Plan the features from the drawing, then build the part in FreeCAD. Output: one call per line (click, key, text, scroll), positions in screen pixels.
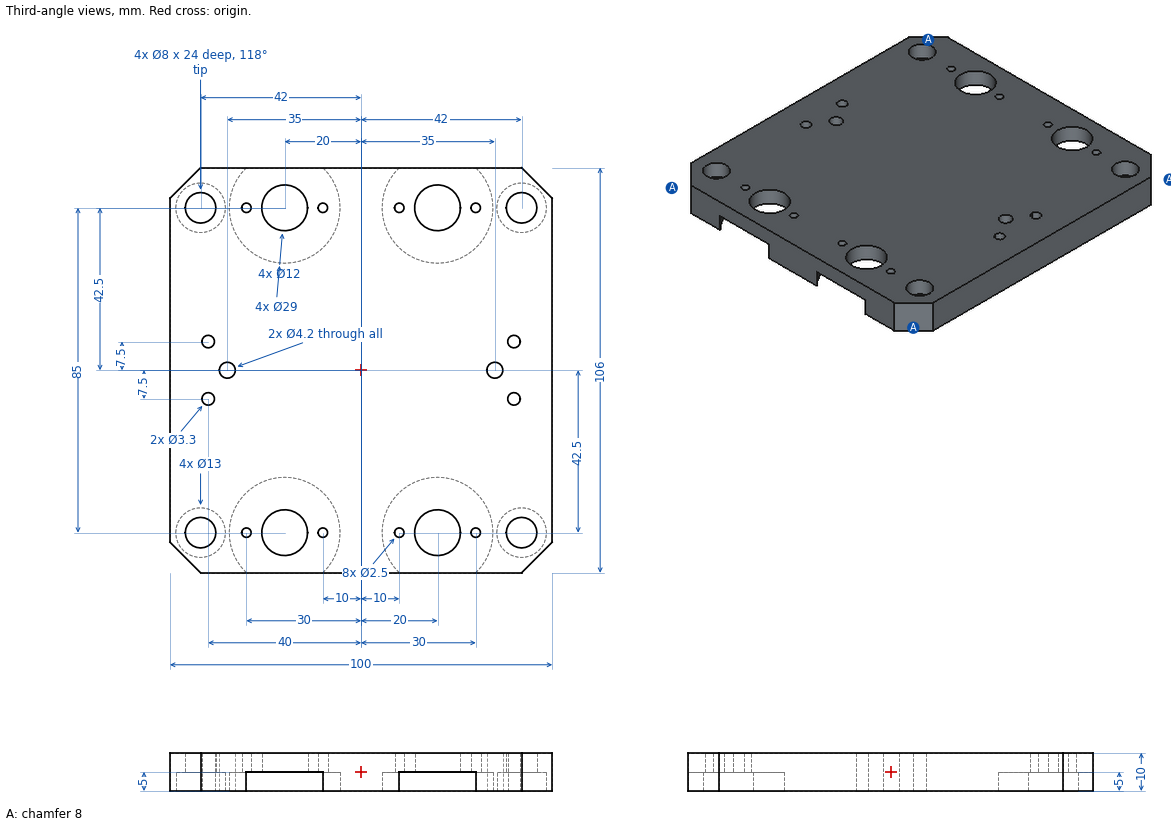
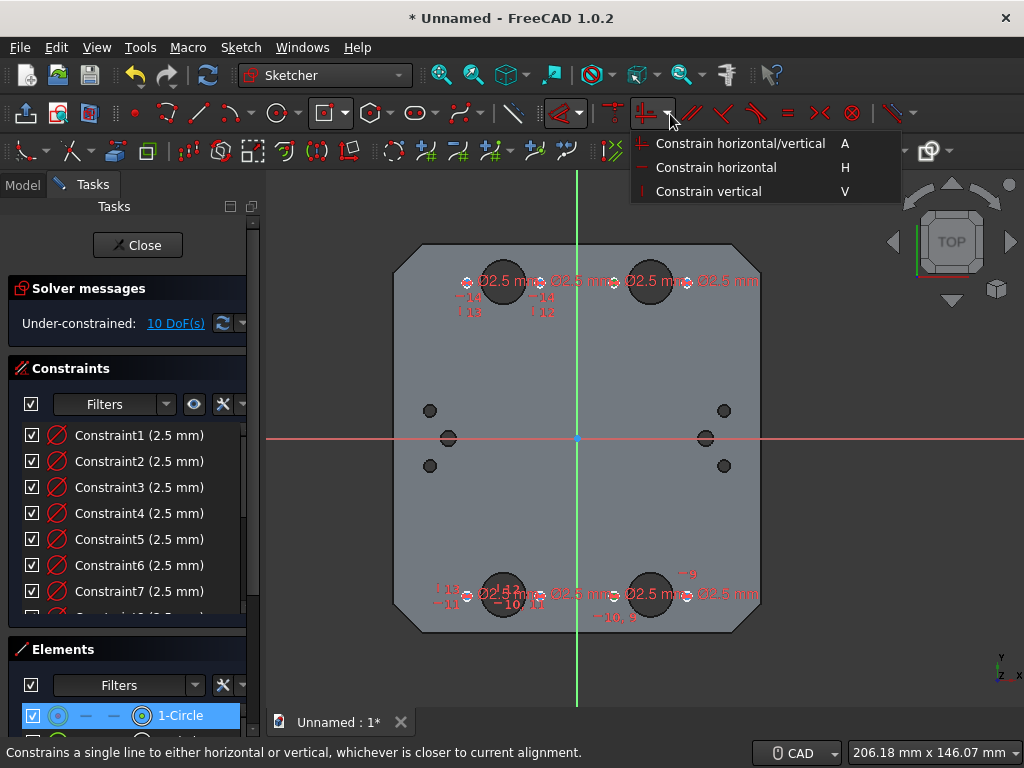
click(766, 191)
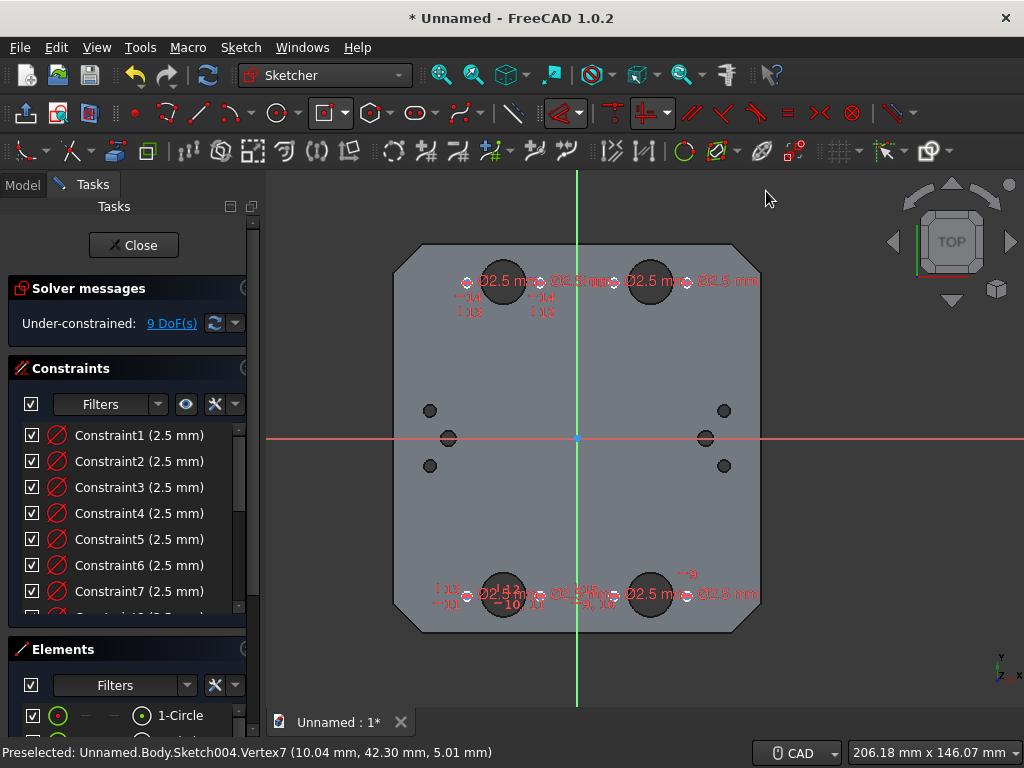
click(540, 283)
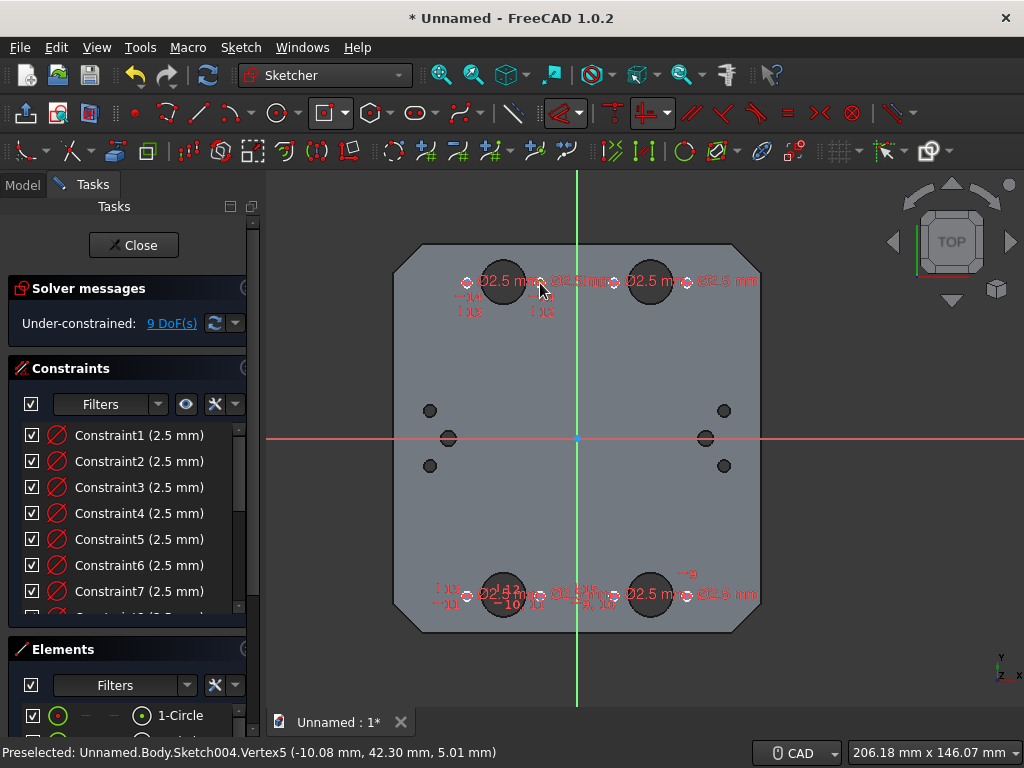
click(614, 283)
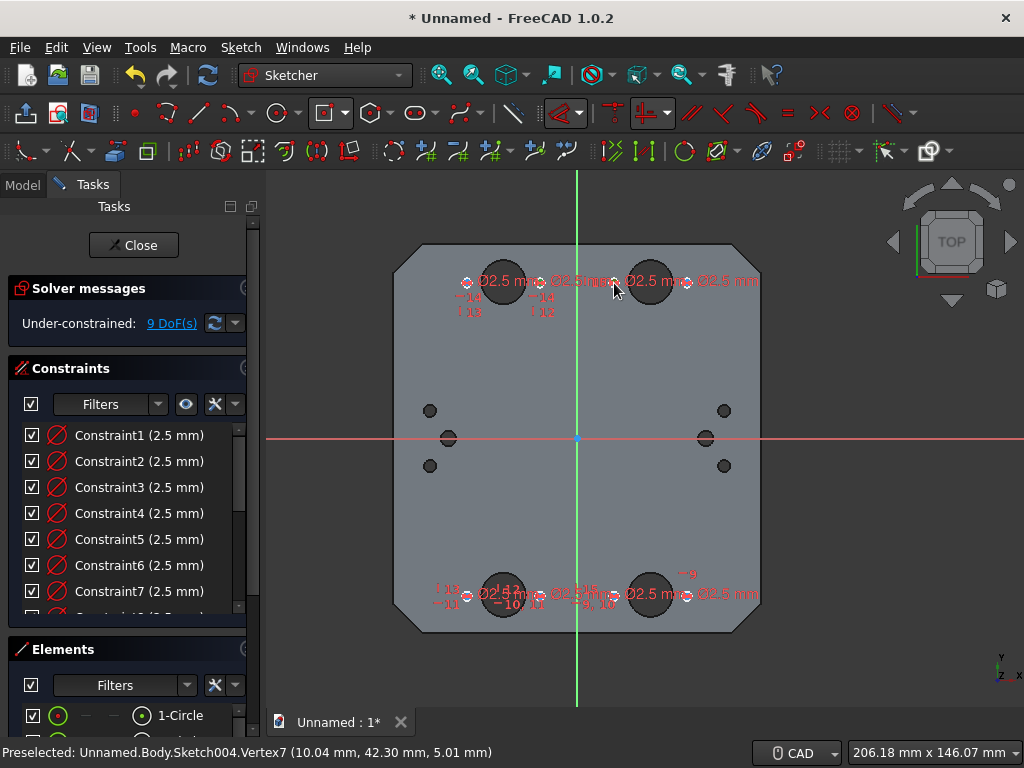
click(670, 114)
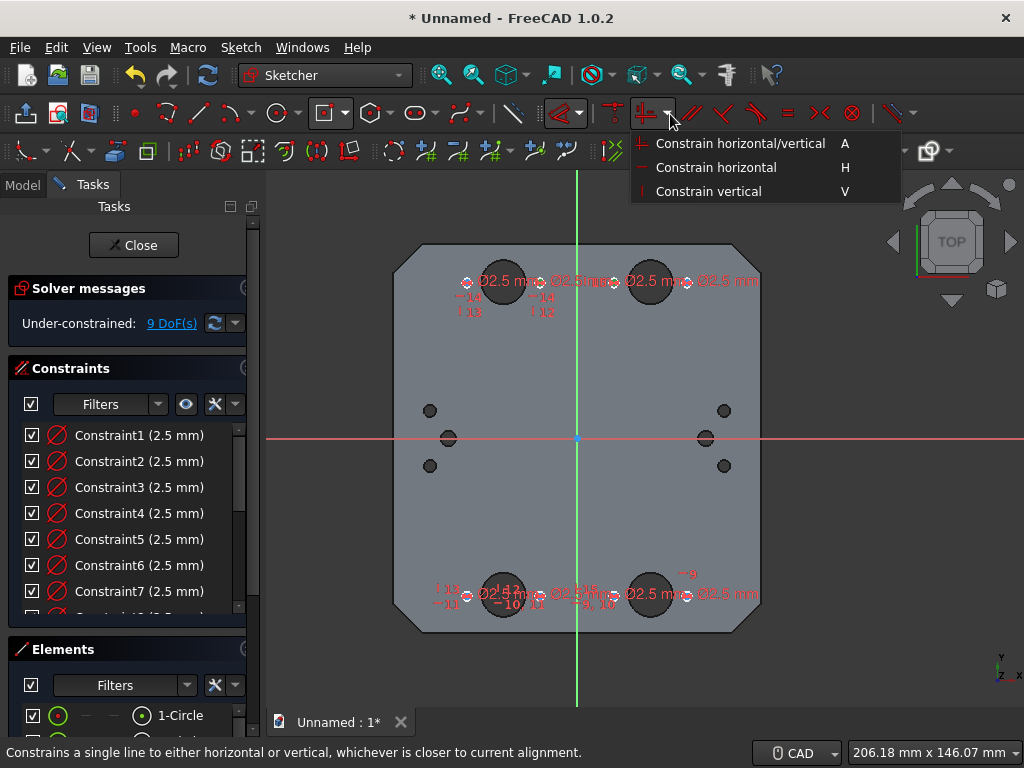
click(766, 167)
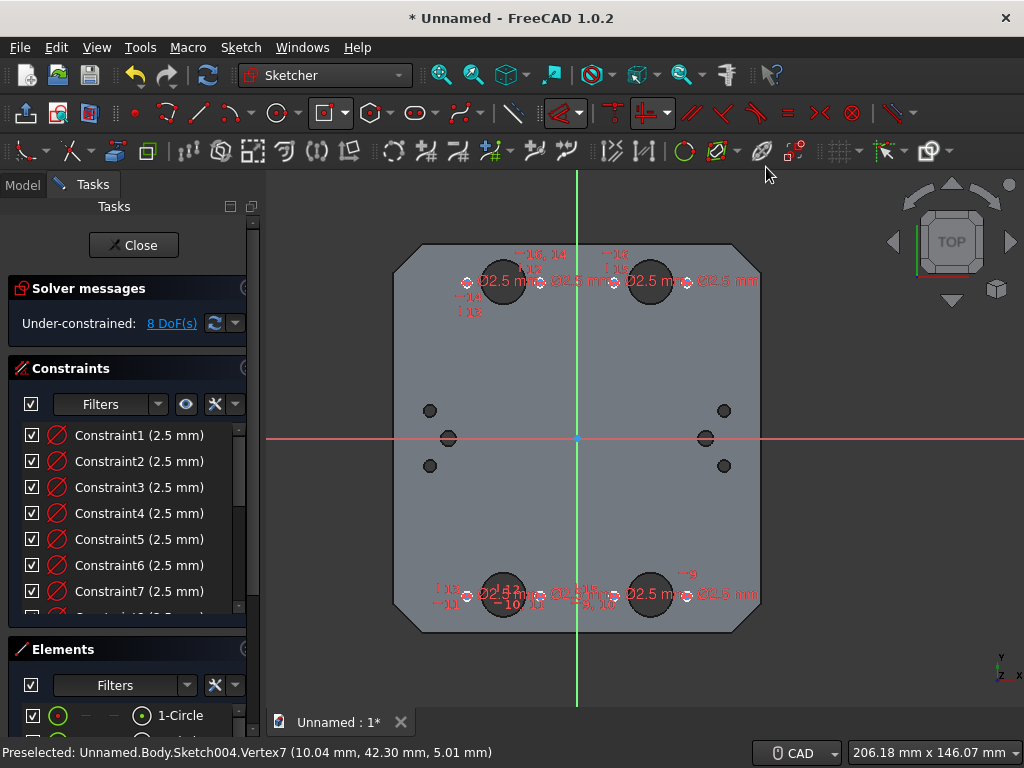
click(687, 596)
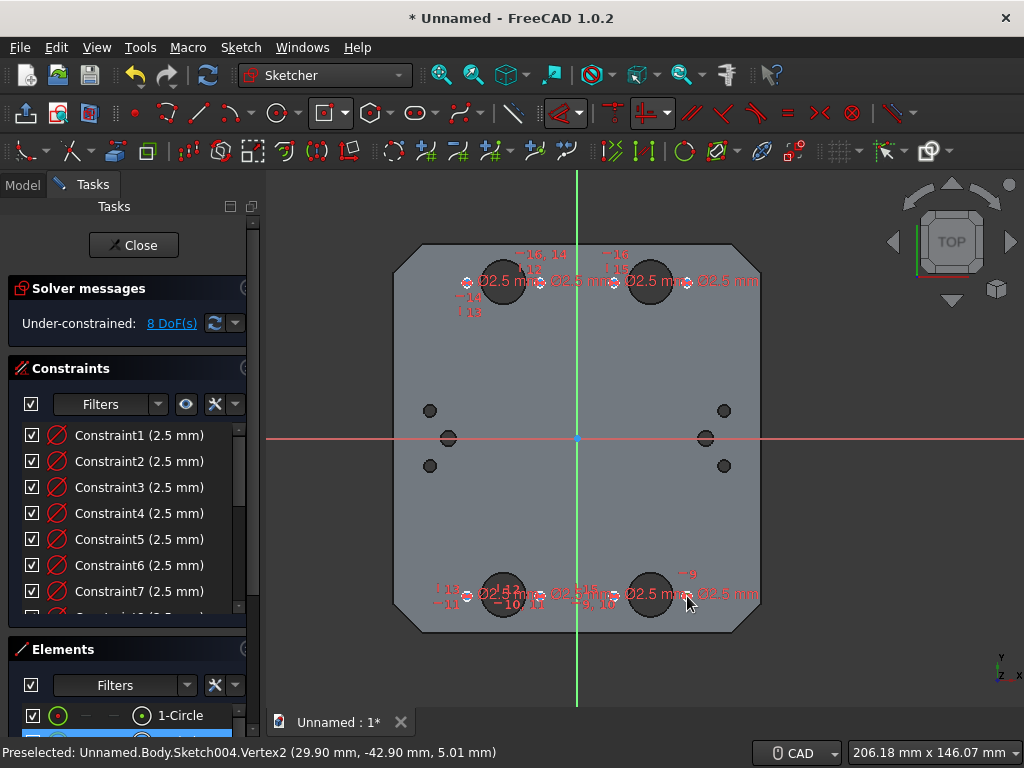
click(687, 283)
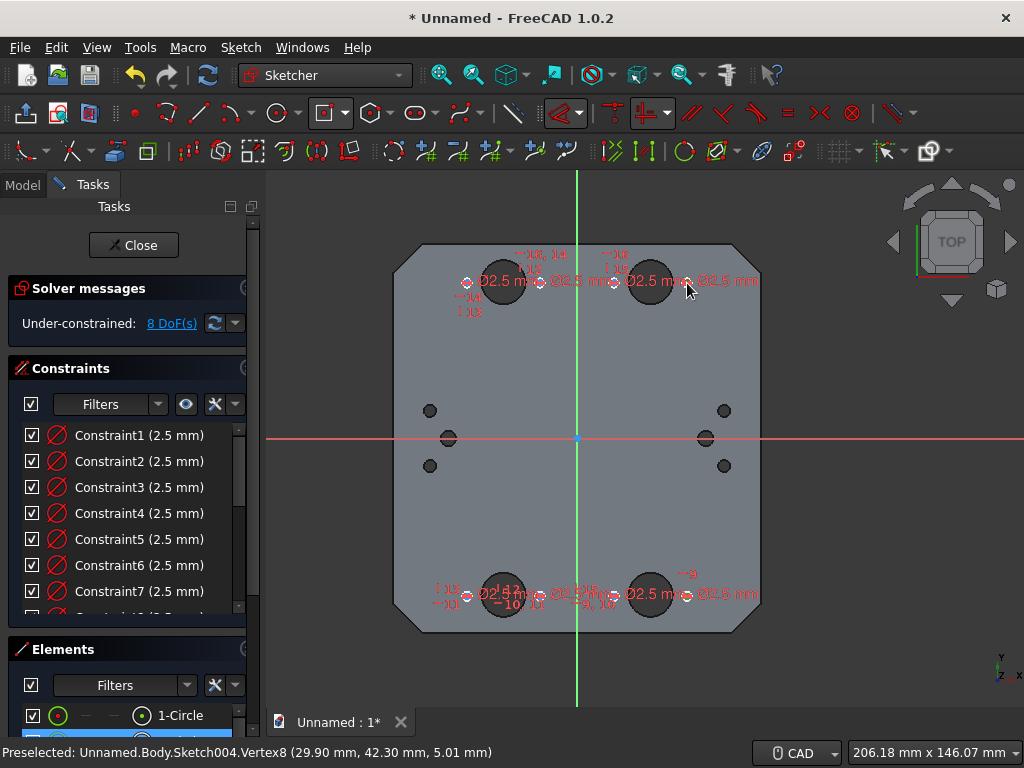
click(670, 114)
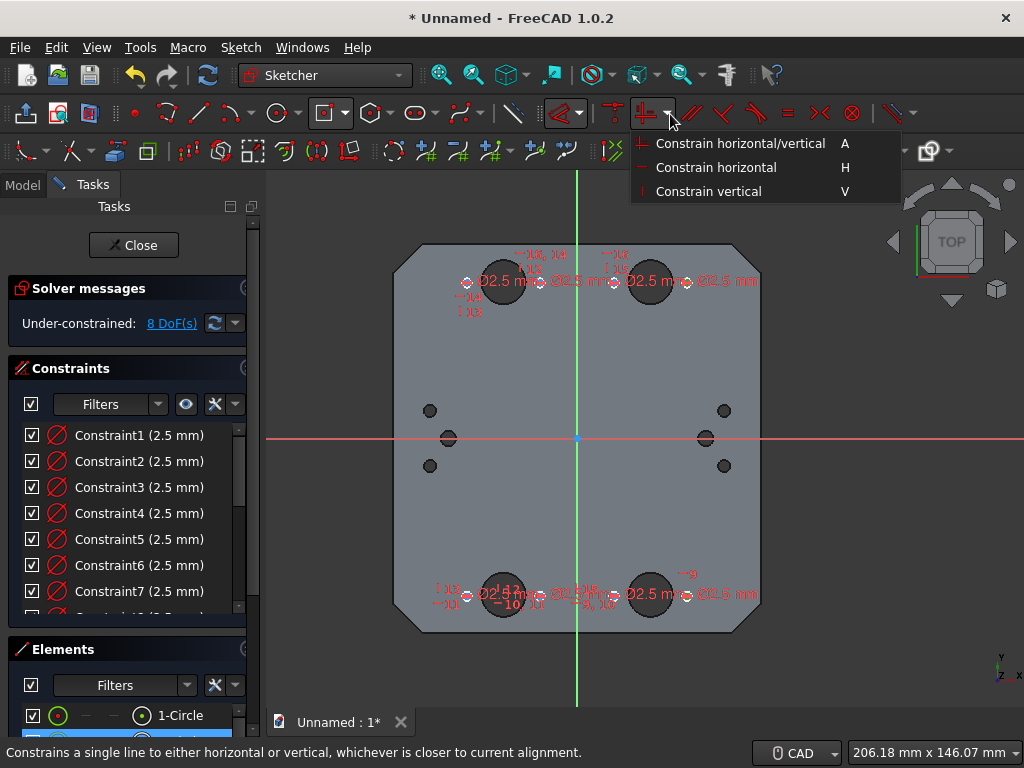
click(766, 191)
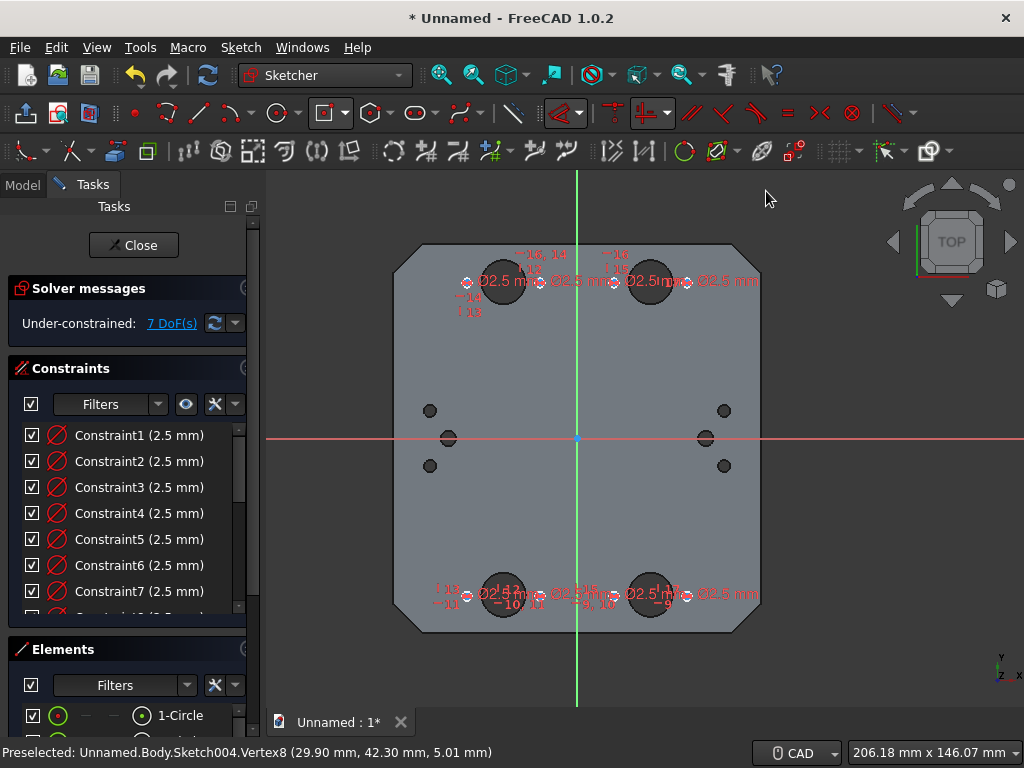
click(614, 283)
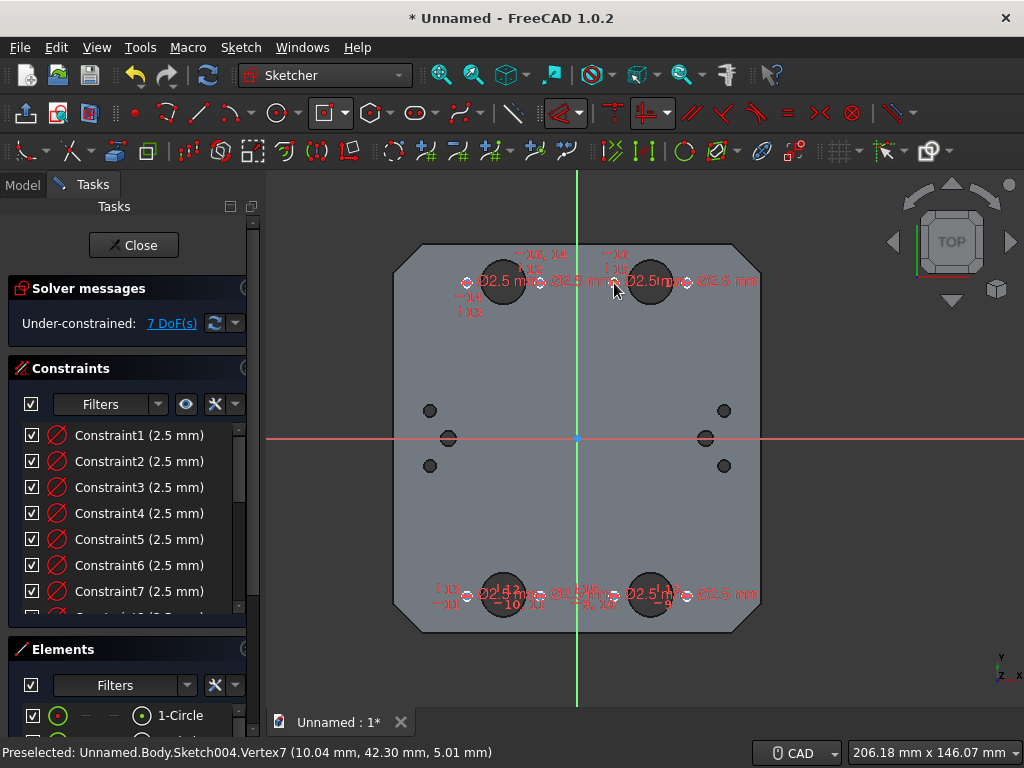
click(687, 283)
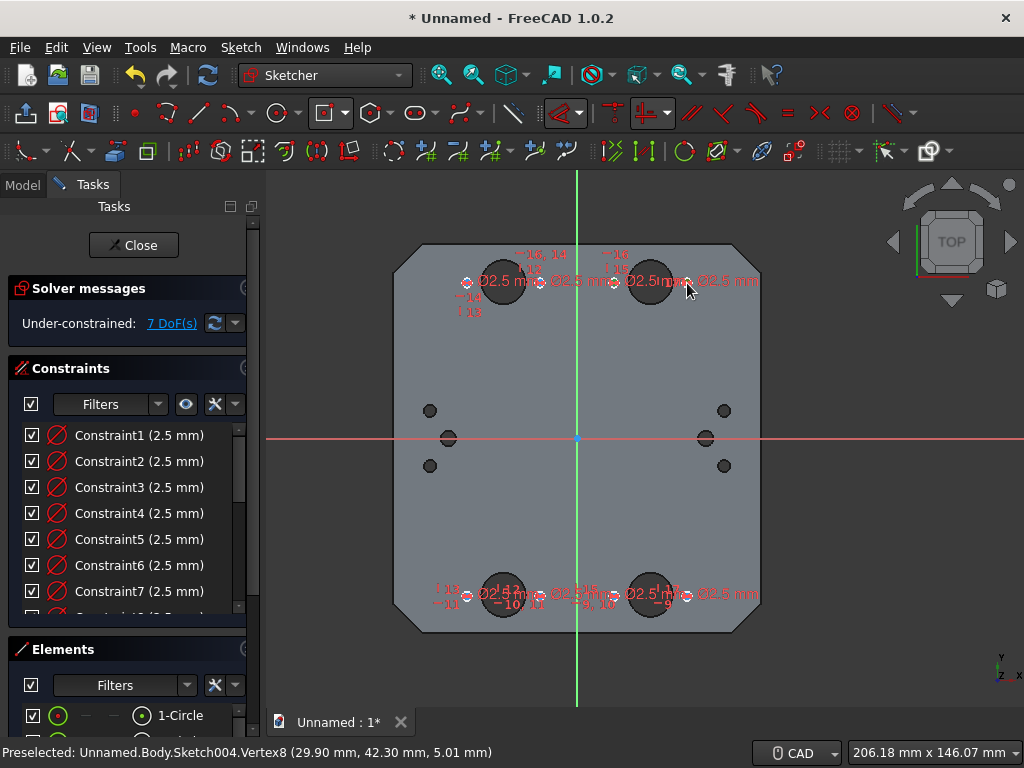
key(h)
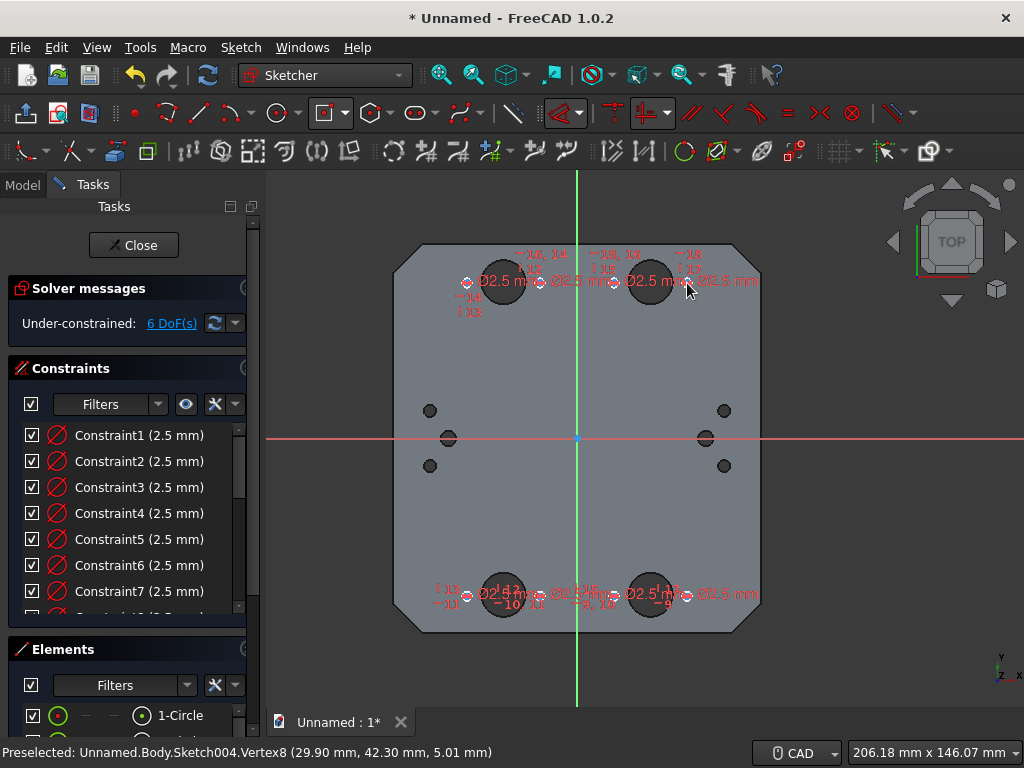
click(614, 596)